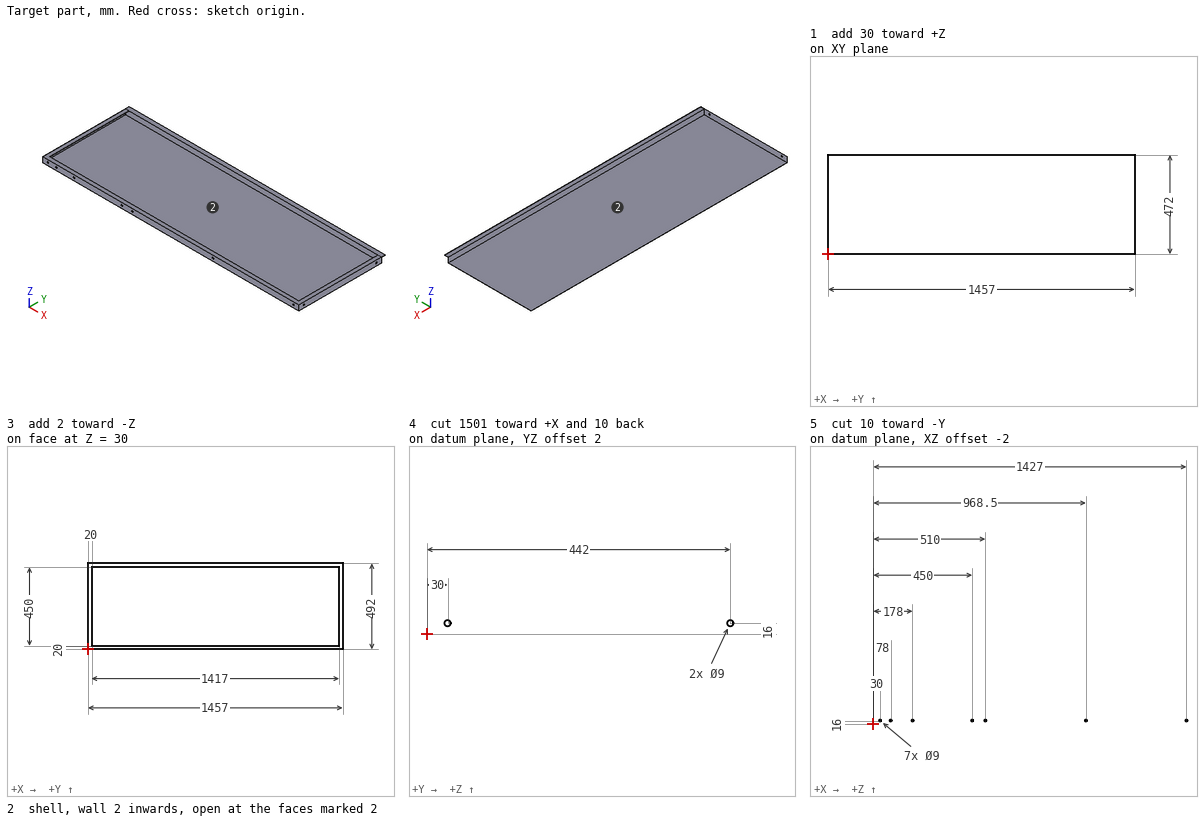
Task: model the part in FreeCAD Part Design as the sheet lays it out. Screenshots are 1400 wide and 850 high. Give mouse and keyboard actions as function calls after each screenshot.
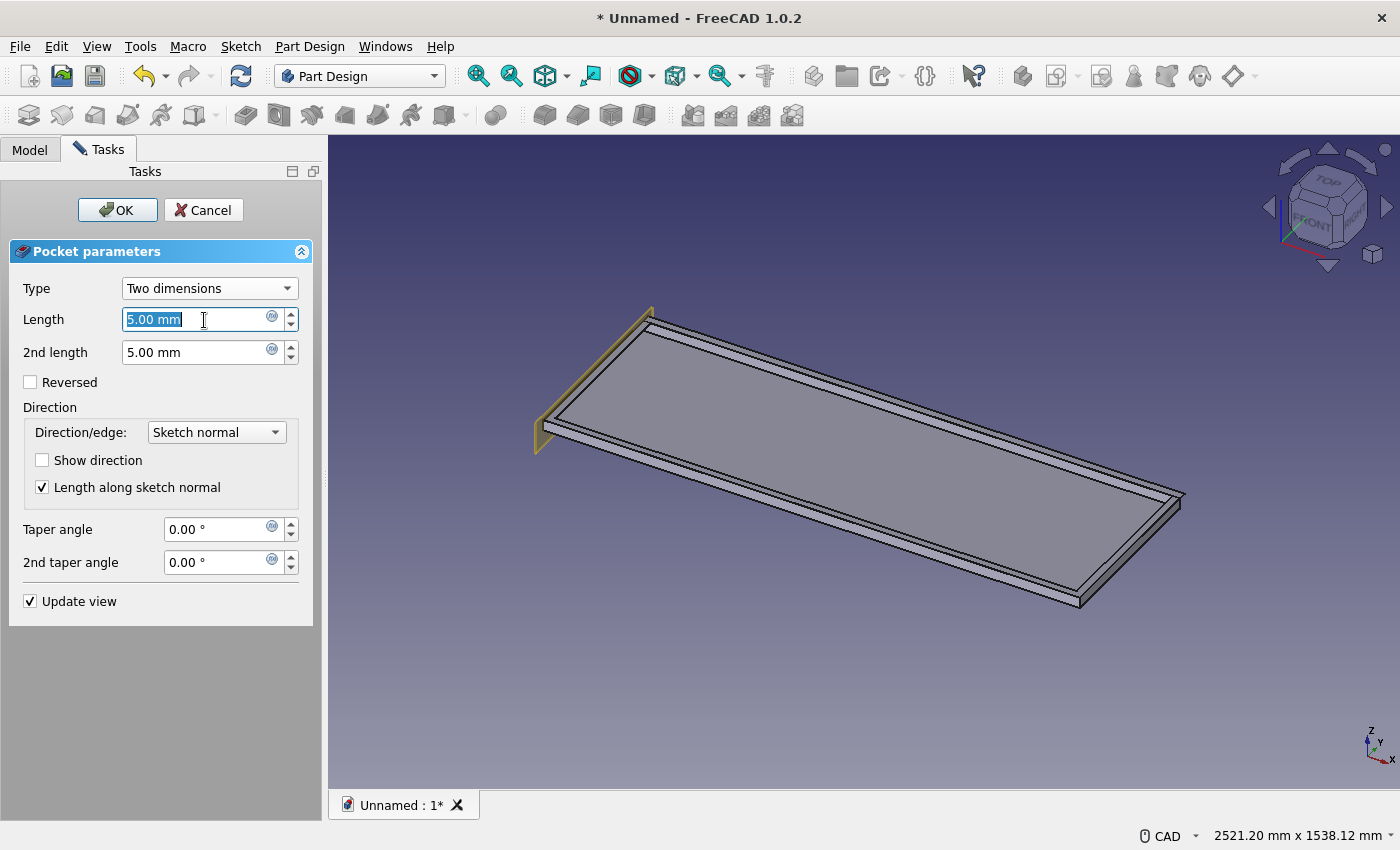
text(1501)
key(Tab)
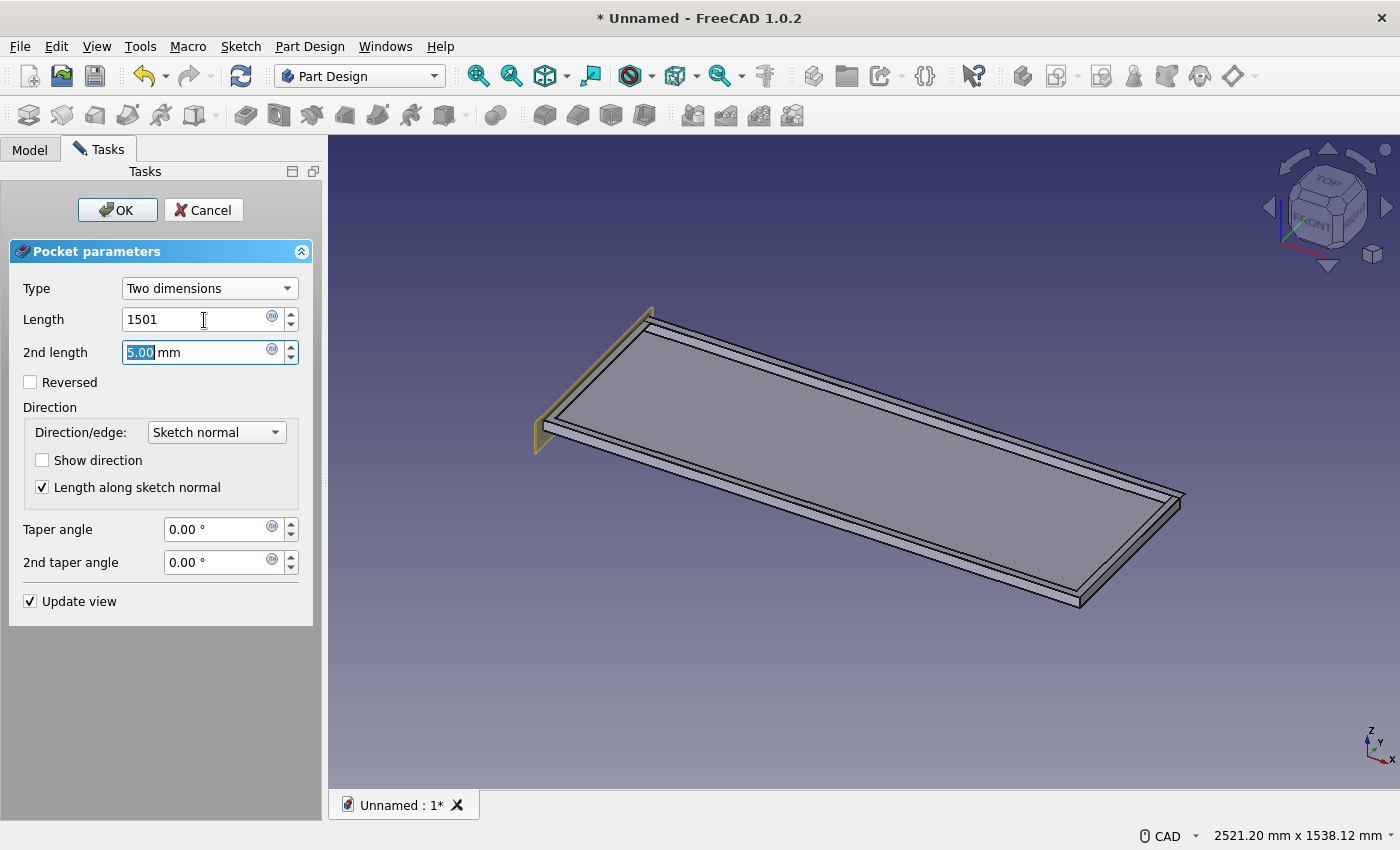
text(10)
key(Tab)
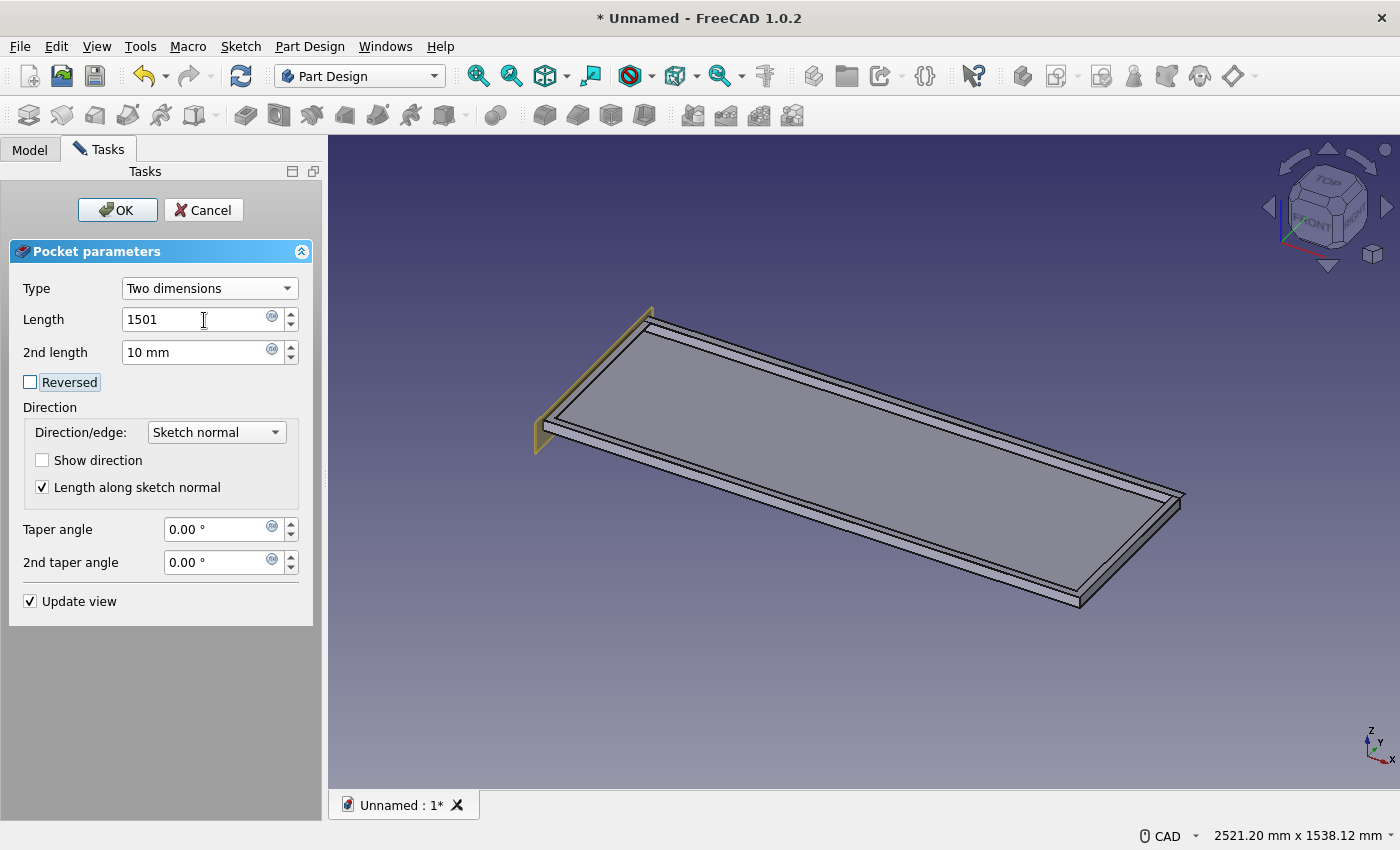
click(31, 382)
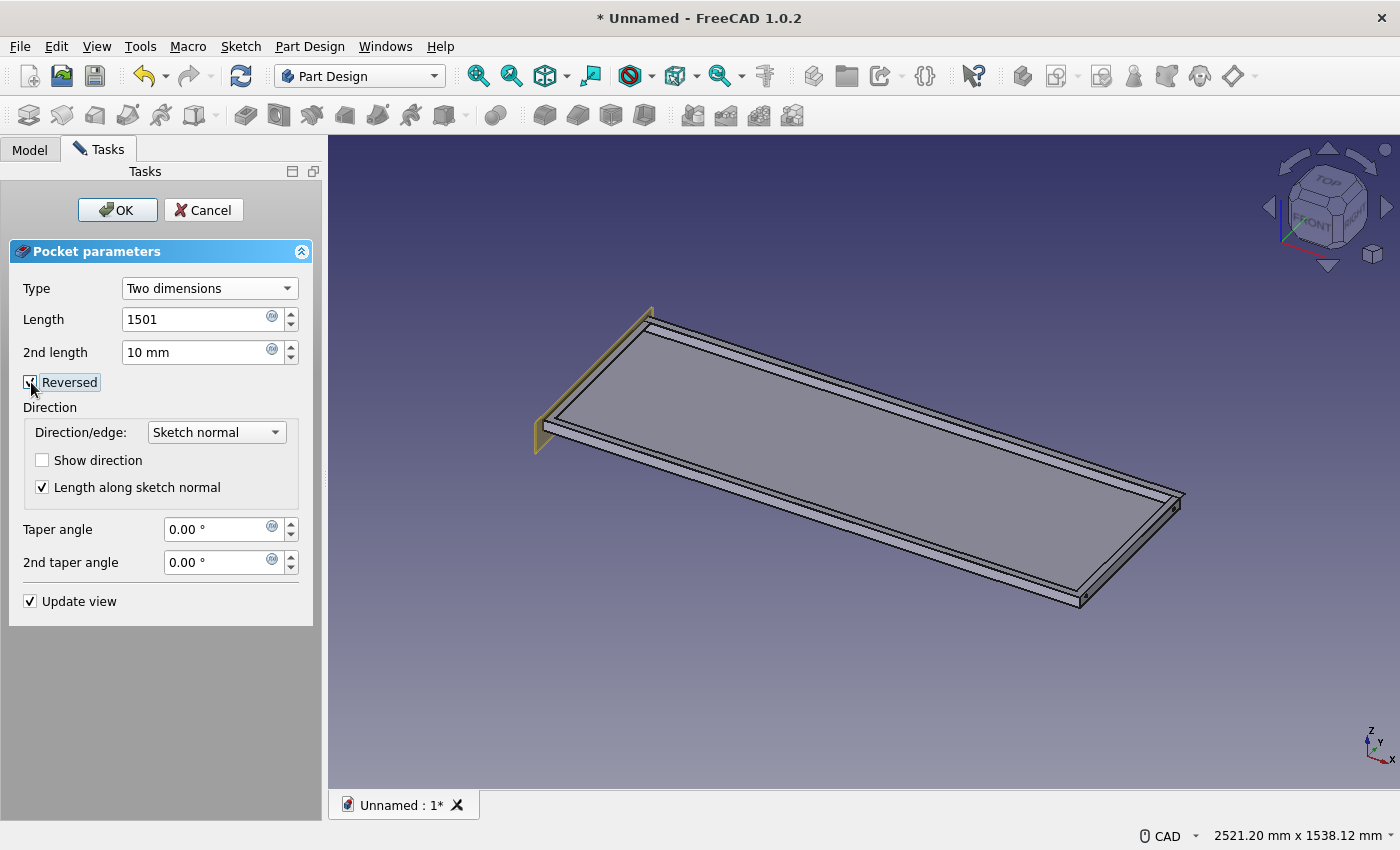
click(118, 210)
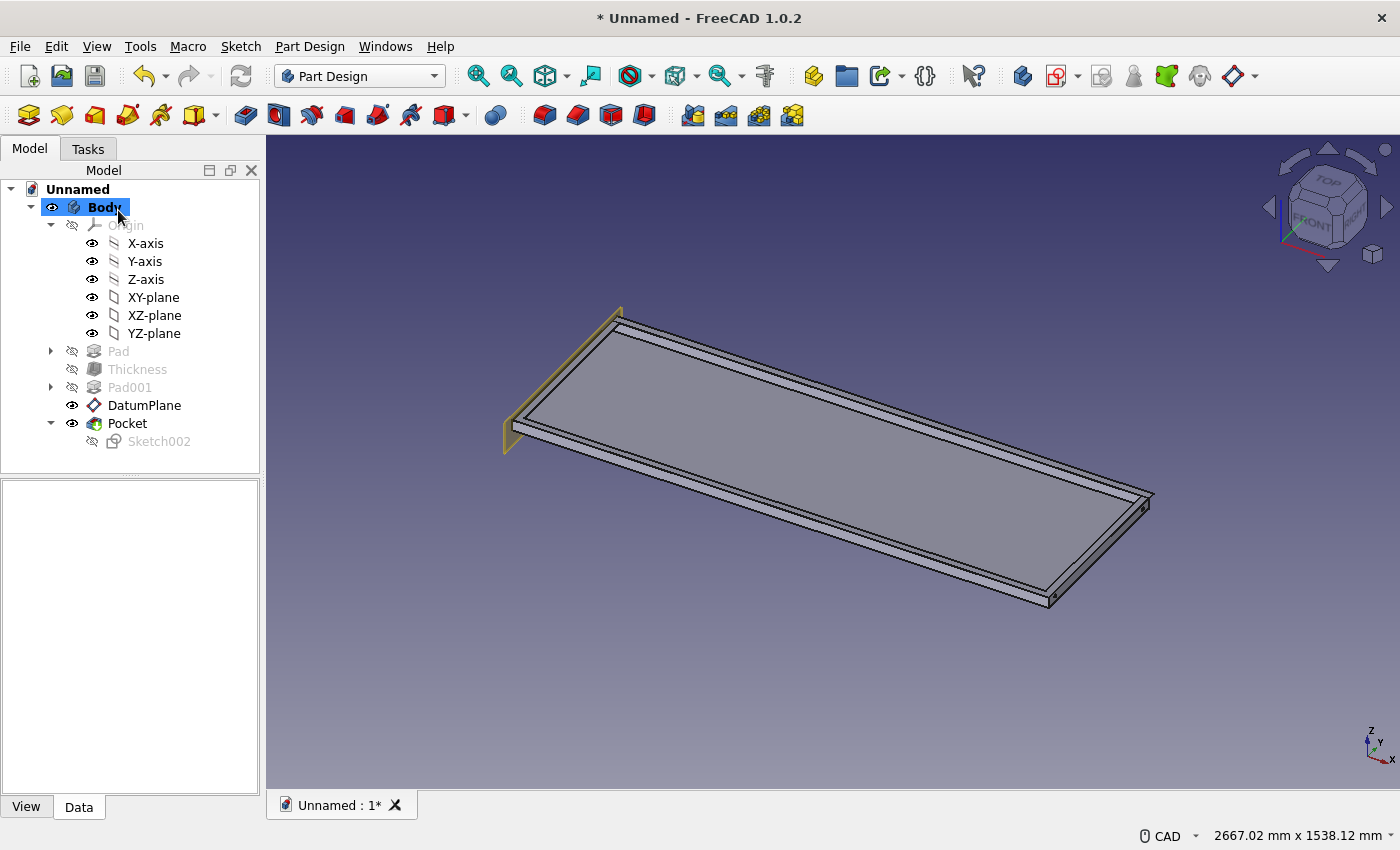
click(117, 405)
key(space)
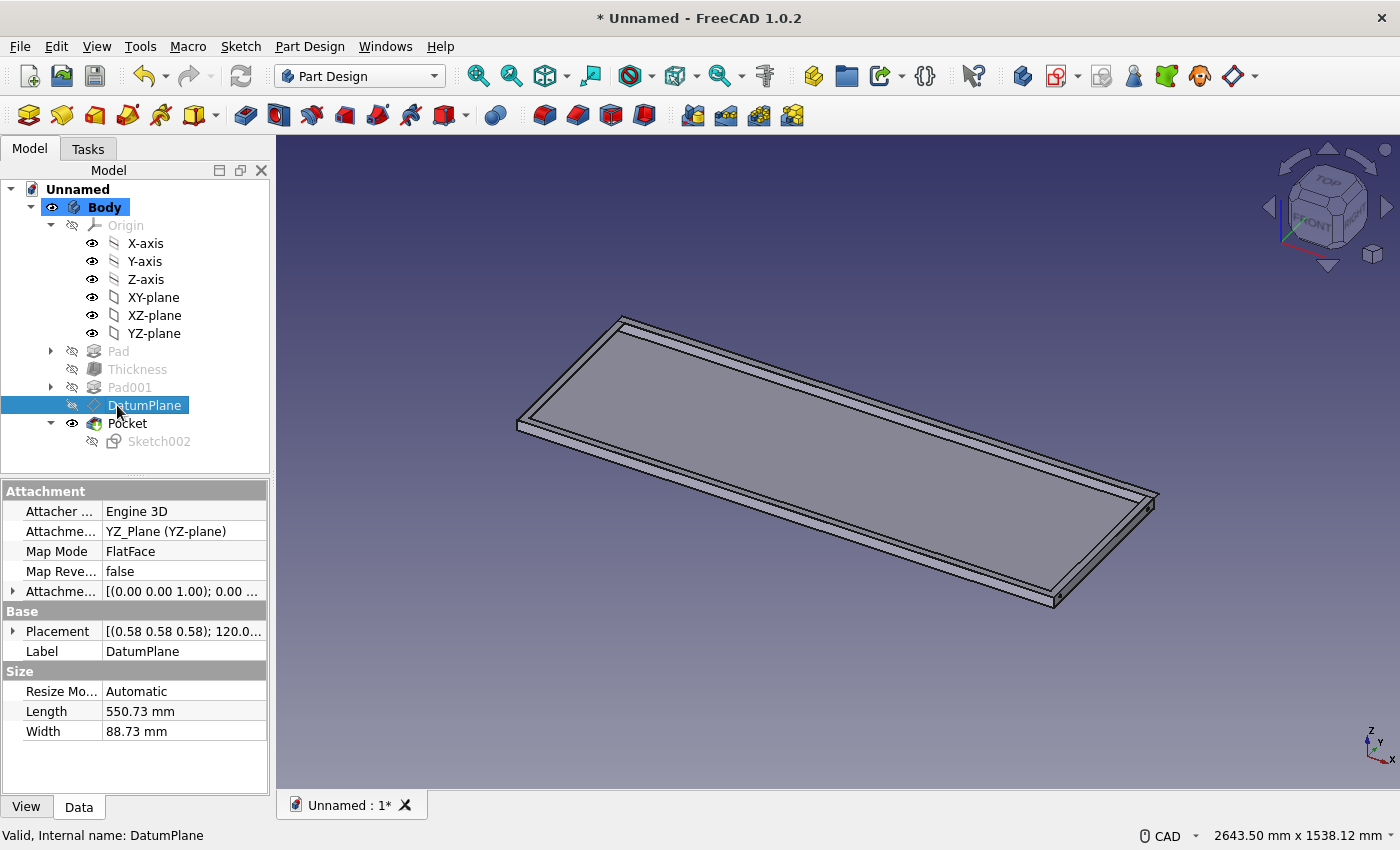
click(137, 315)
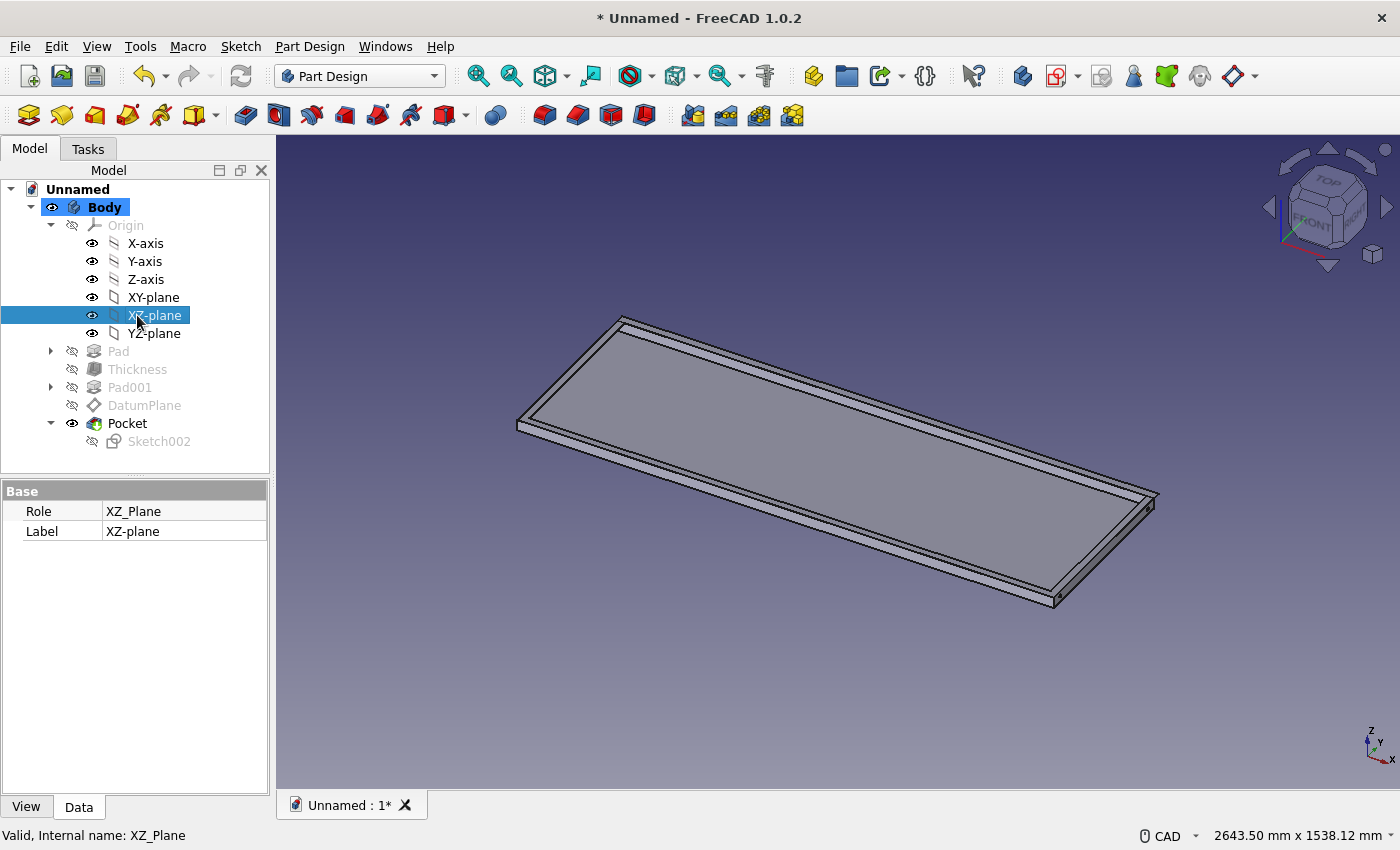
click(1232, 76)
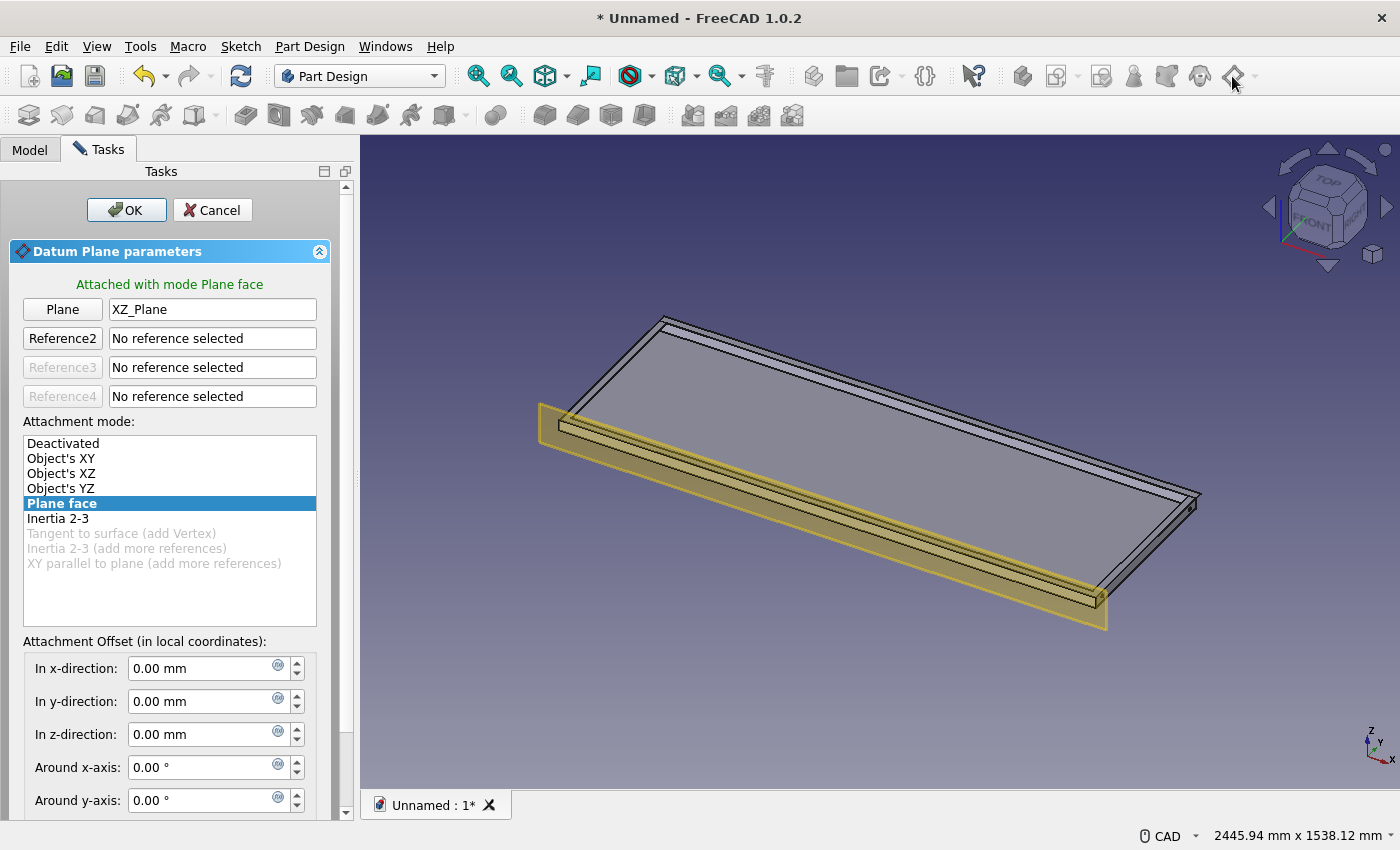
triple_click(210, 734)